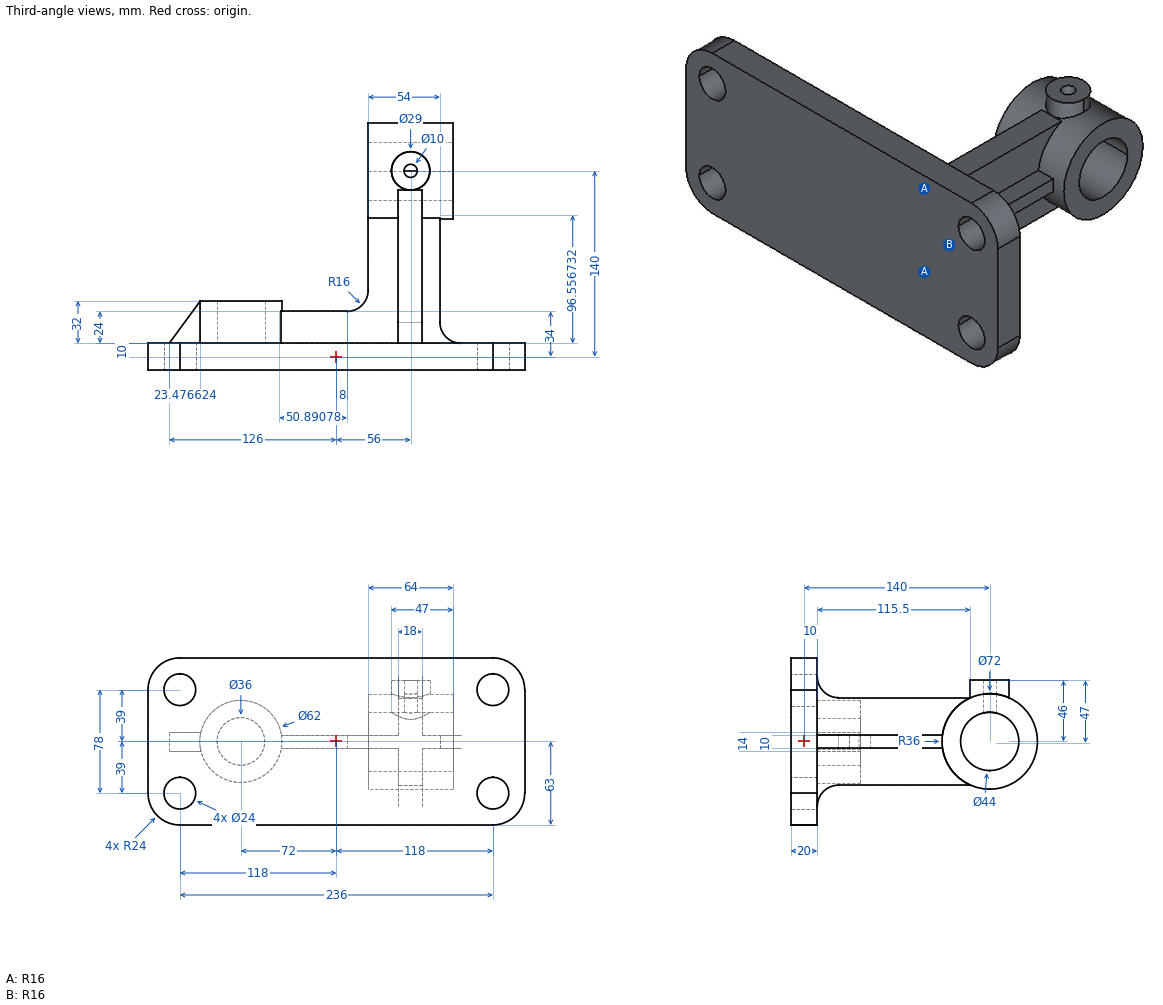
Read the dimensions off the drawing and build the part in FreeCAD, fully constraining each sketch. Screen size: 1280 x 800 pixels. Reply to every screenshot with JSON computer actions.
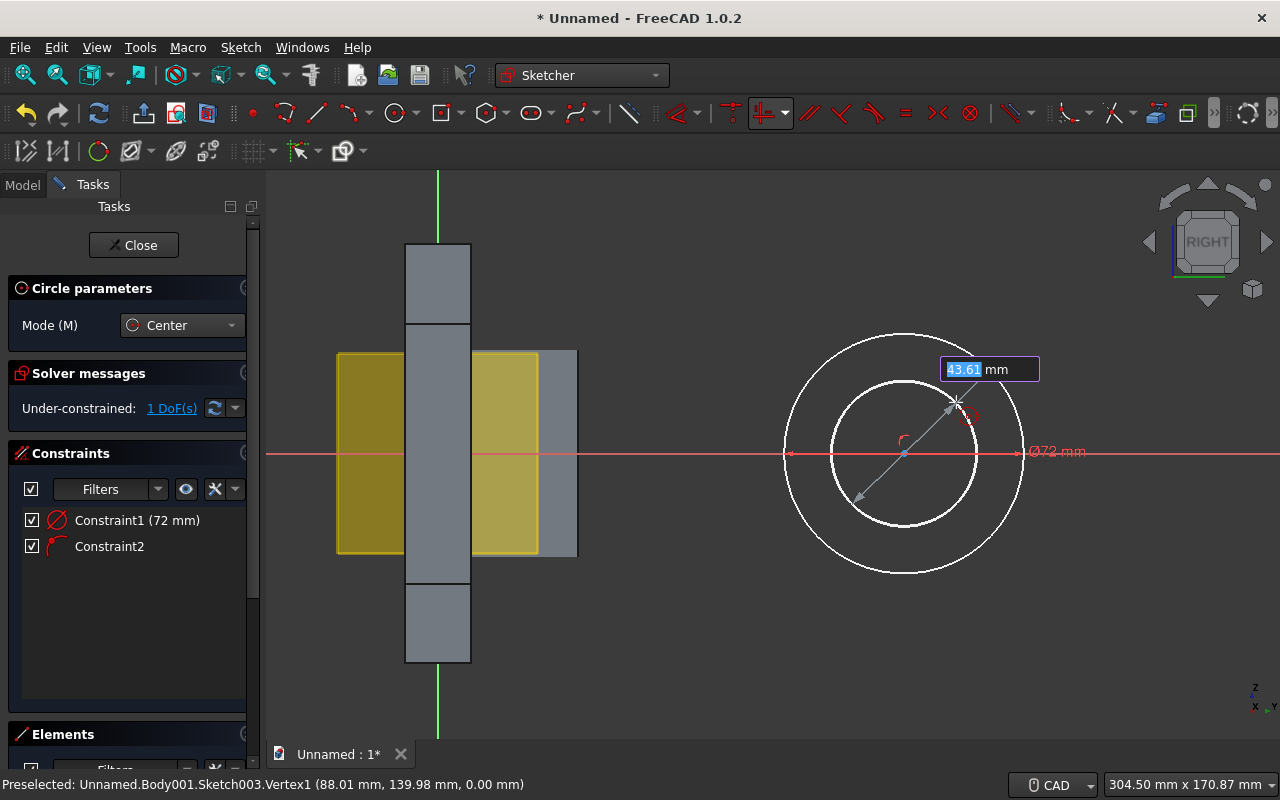
{"action": "type", "text": "44"}
{"action": "key", "text": "Return"}
{"action": "key", "text": "Escape"}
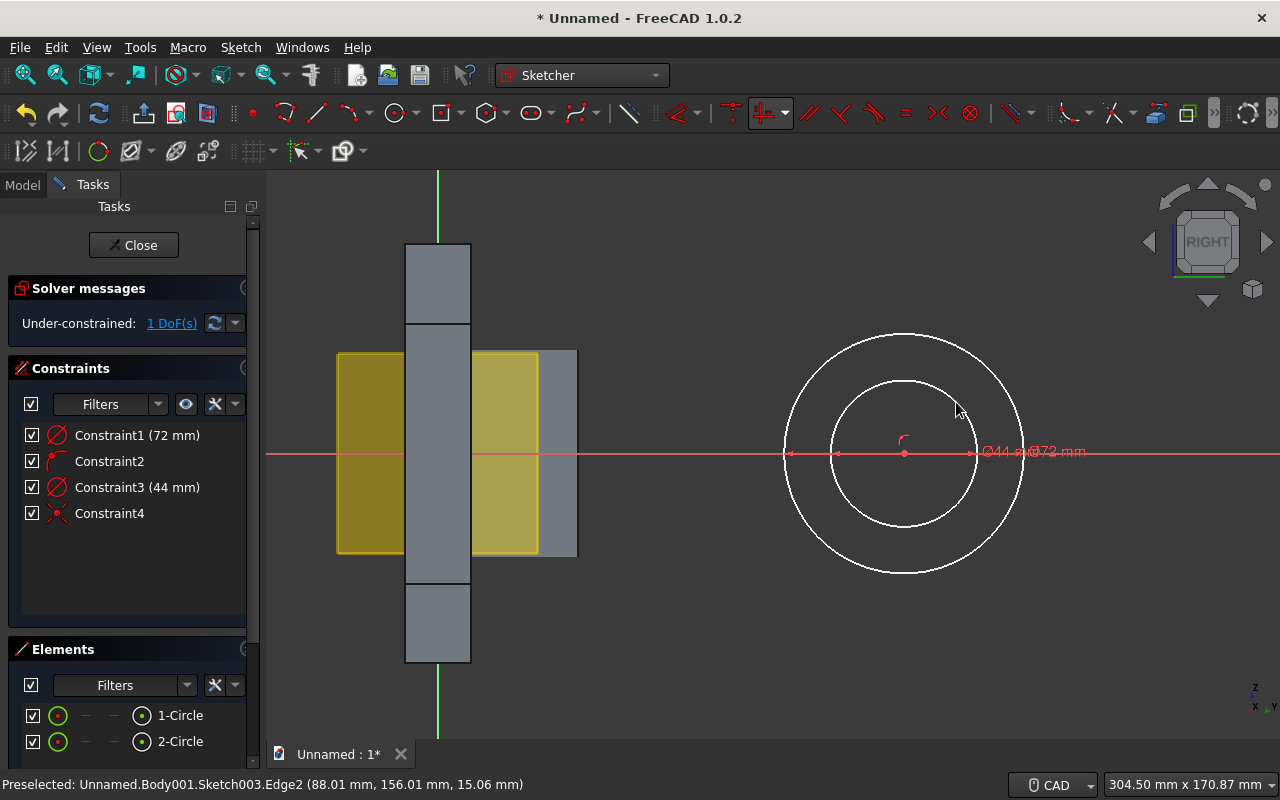
{"action": "left_click", "coordinate": [676, 114]}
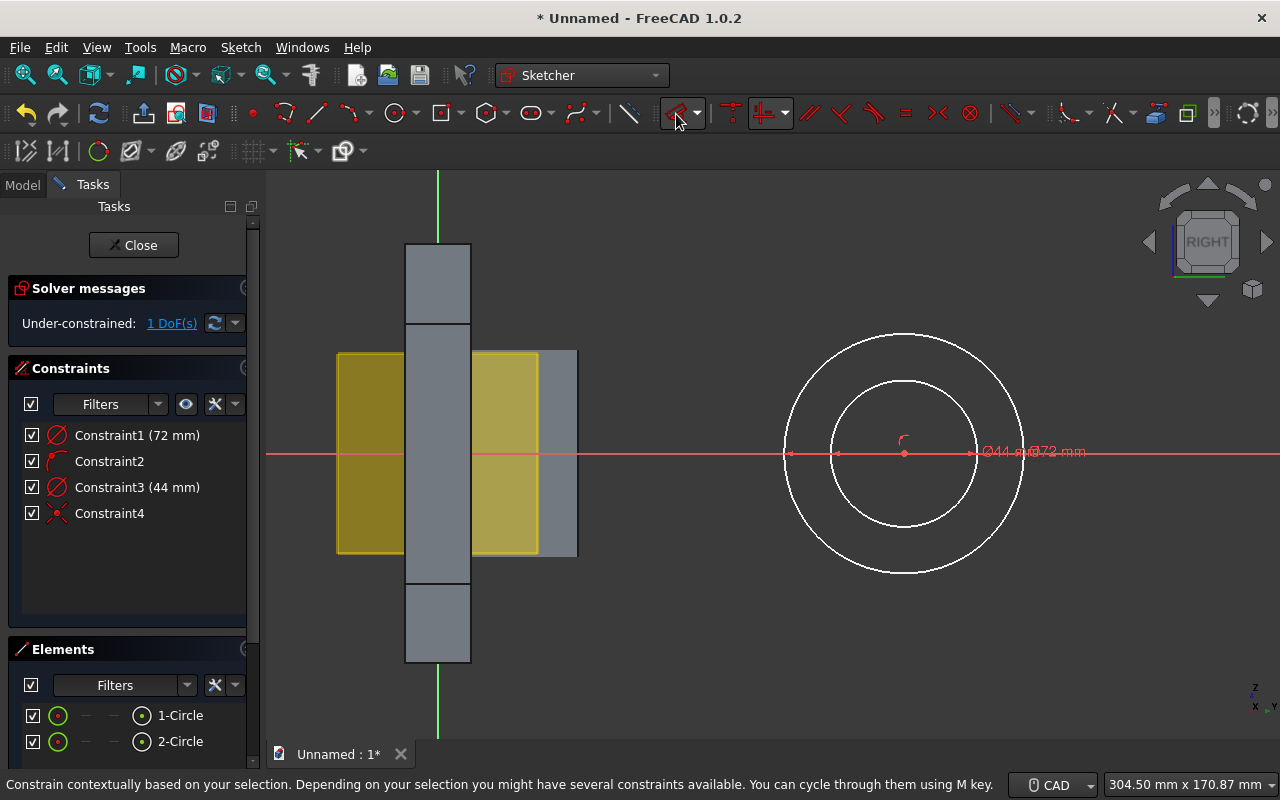
{"action": "left_click", "coordinate": [904, 454]}
{"action": "left_click", "coordinate": [671, 488]}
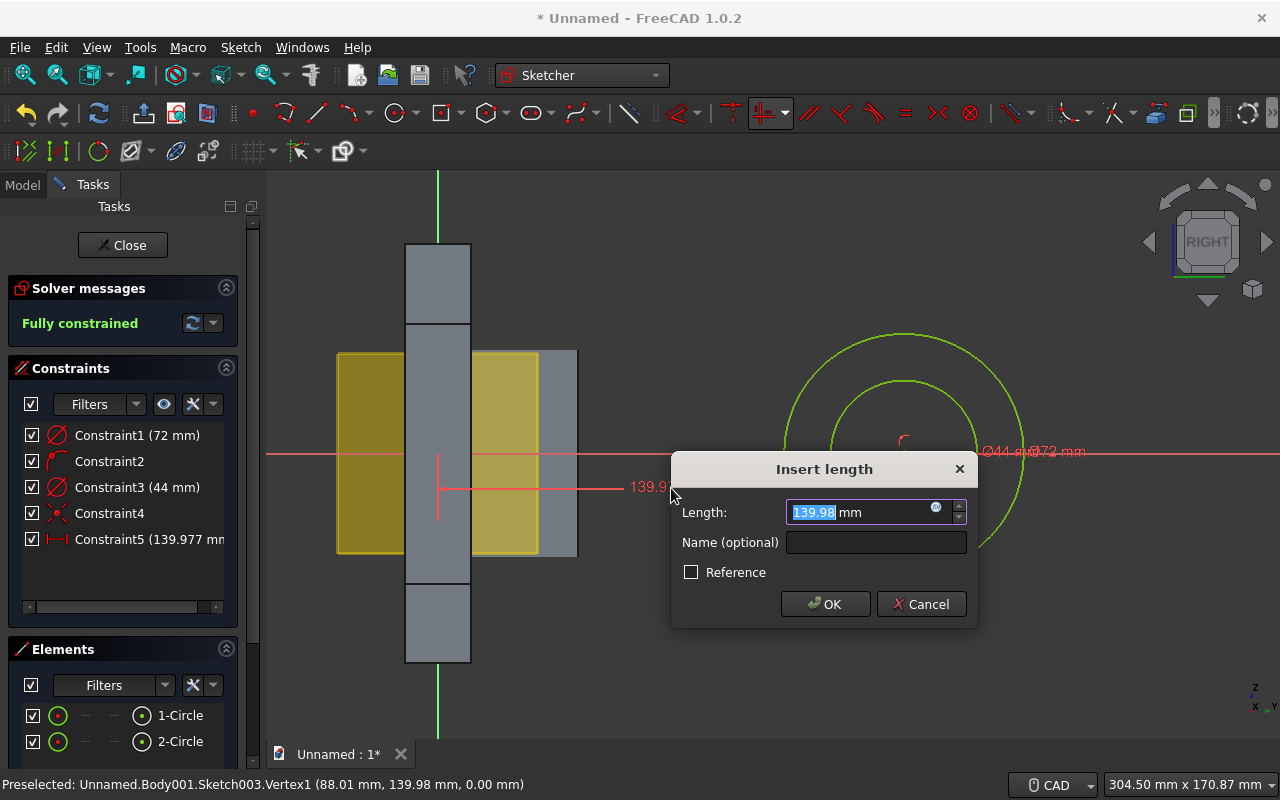
{"action": "type", "text": "140"}
{"action": "key", "text": "Return"}
{"action": "key", "text": "Escape"}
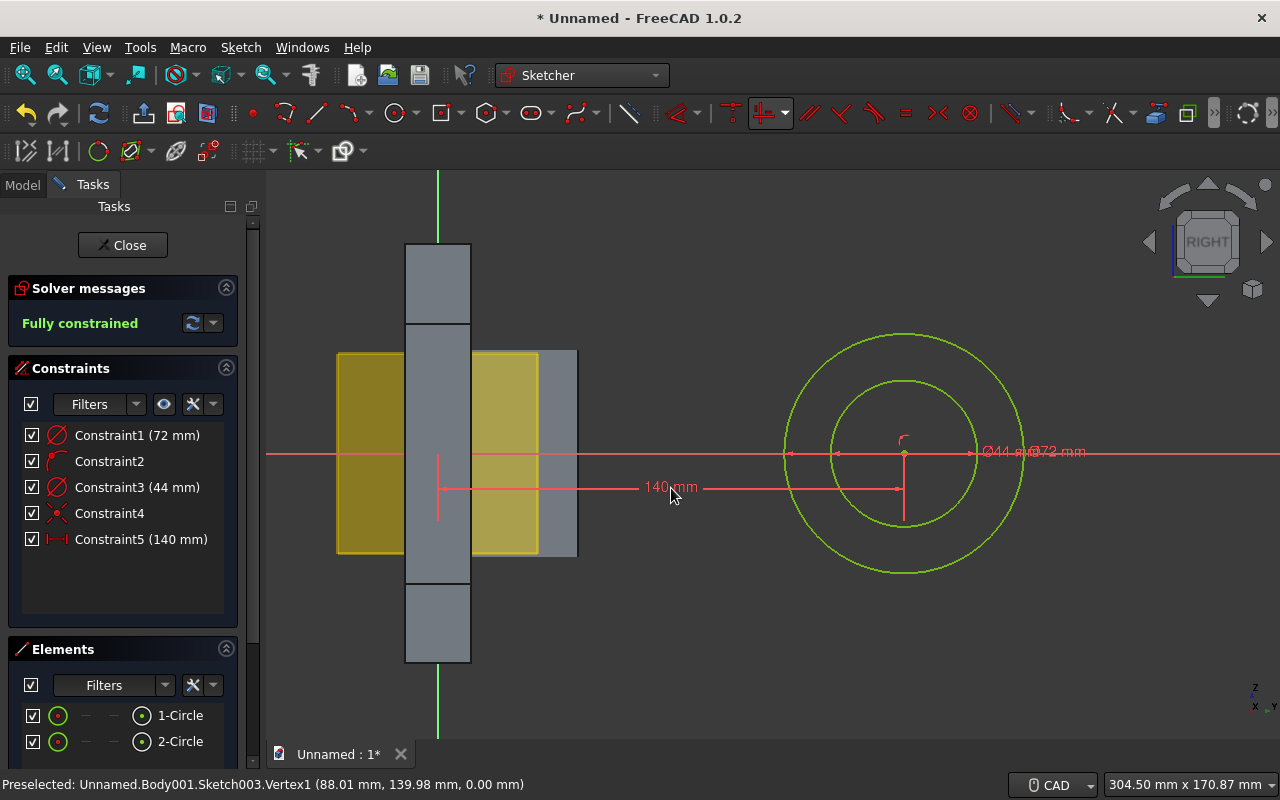
{"action": "left_click", "coordinate": [123, 245]}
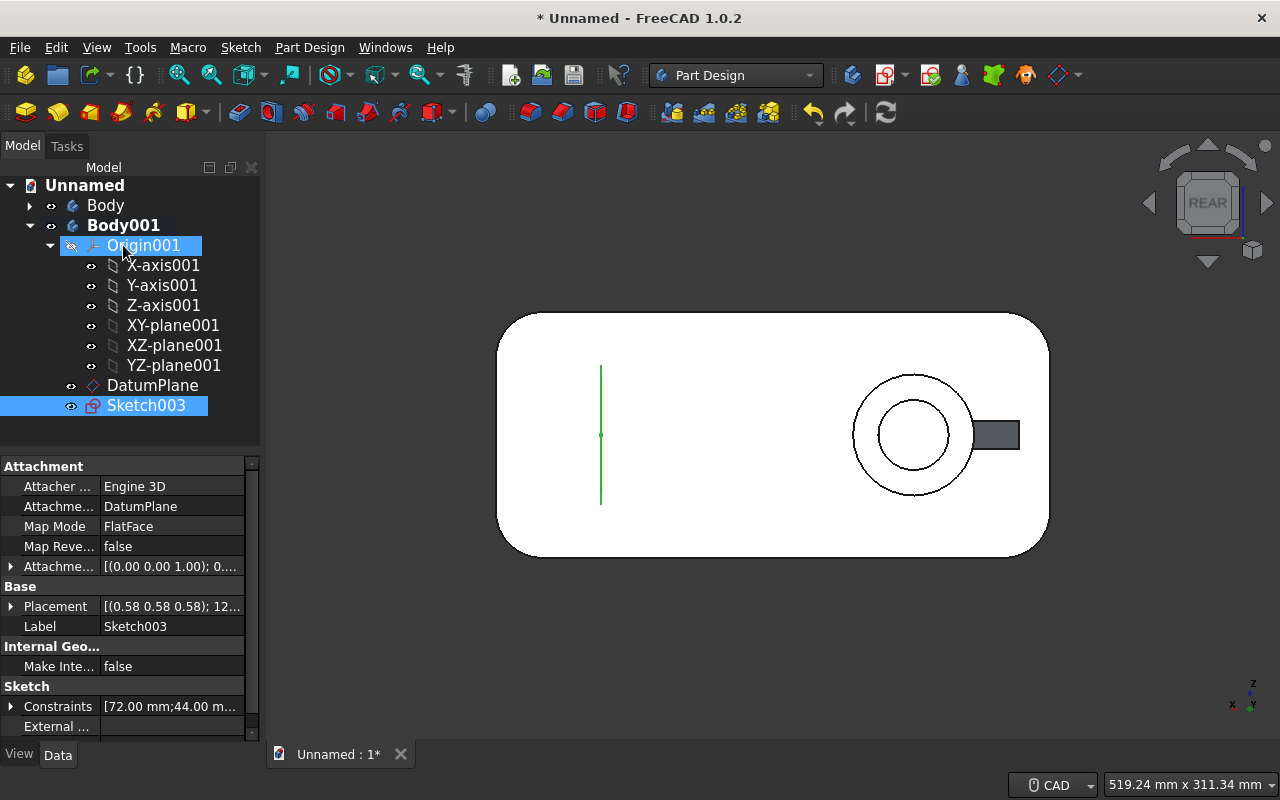
{"action": "left_click", "coordinate": [26, 112]}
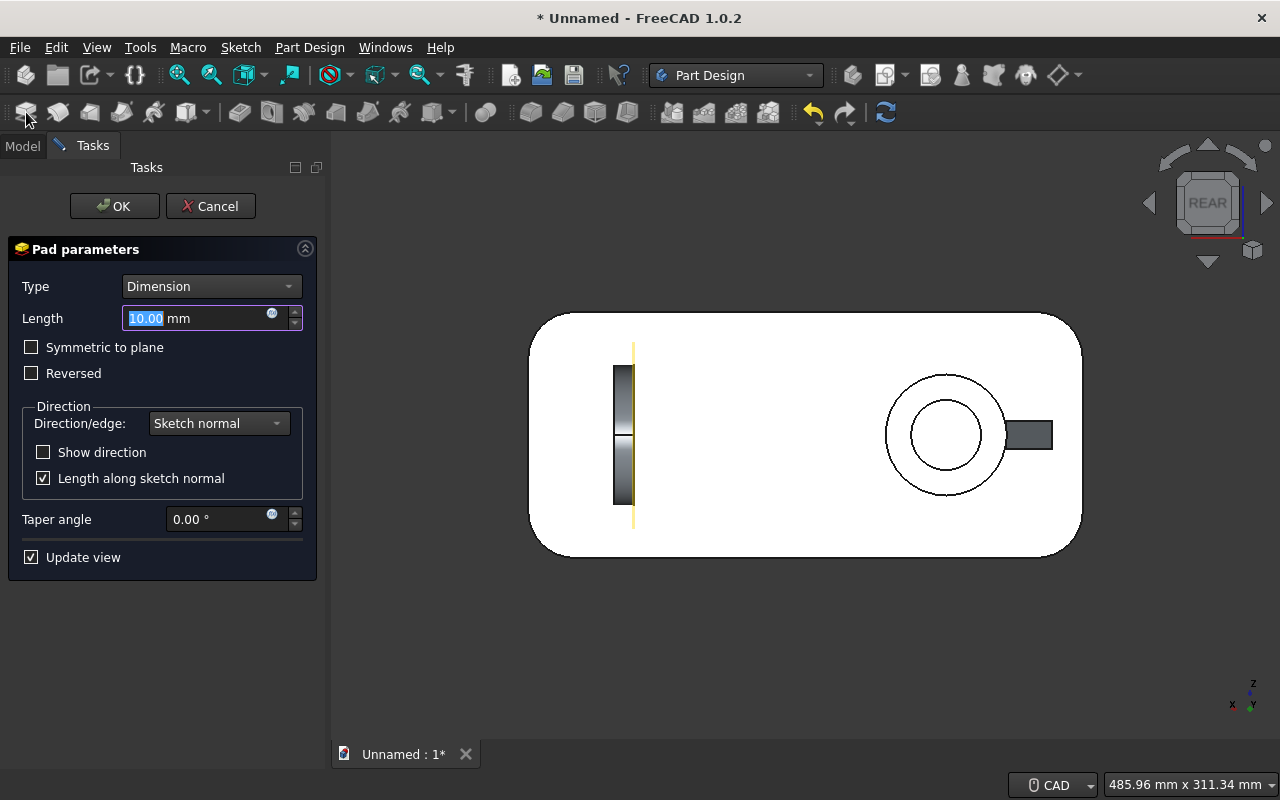
{"action": "type", "text": "64"}
{"action": "key", "text": "Tab"}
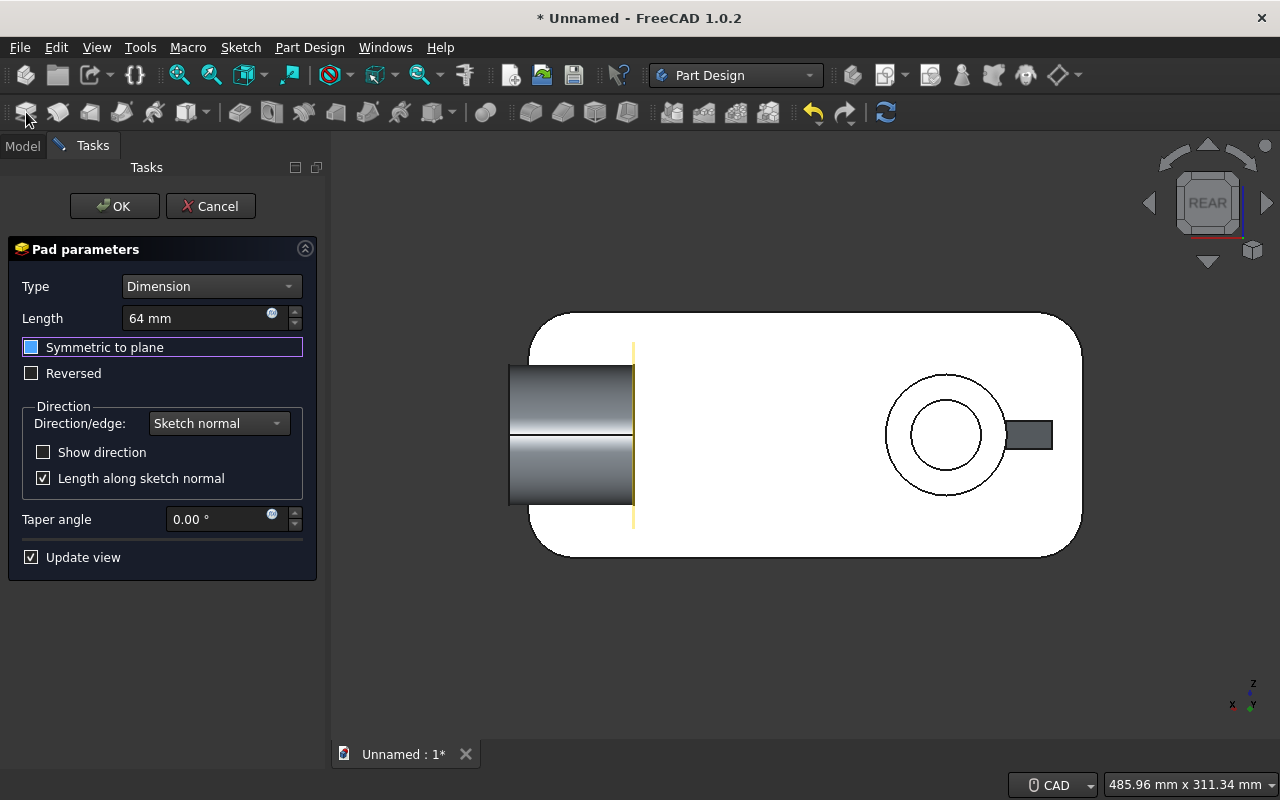
{"action": "left_click", "coordinate": [30, 373]}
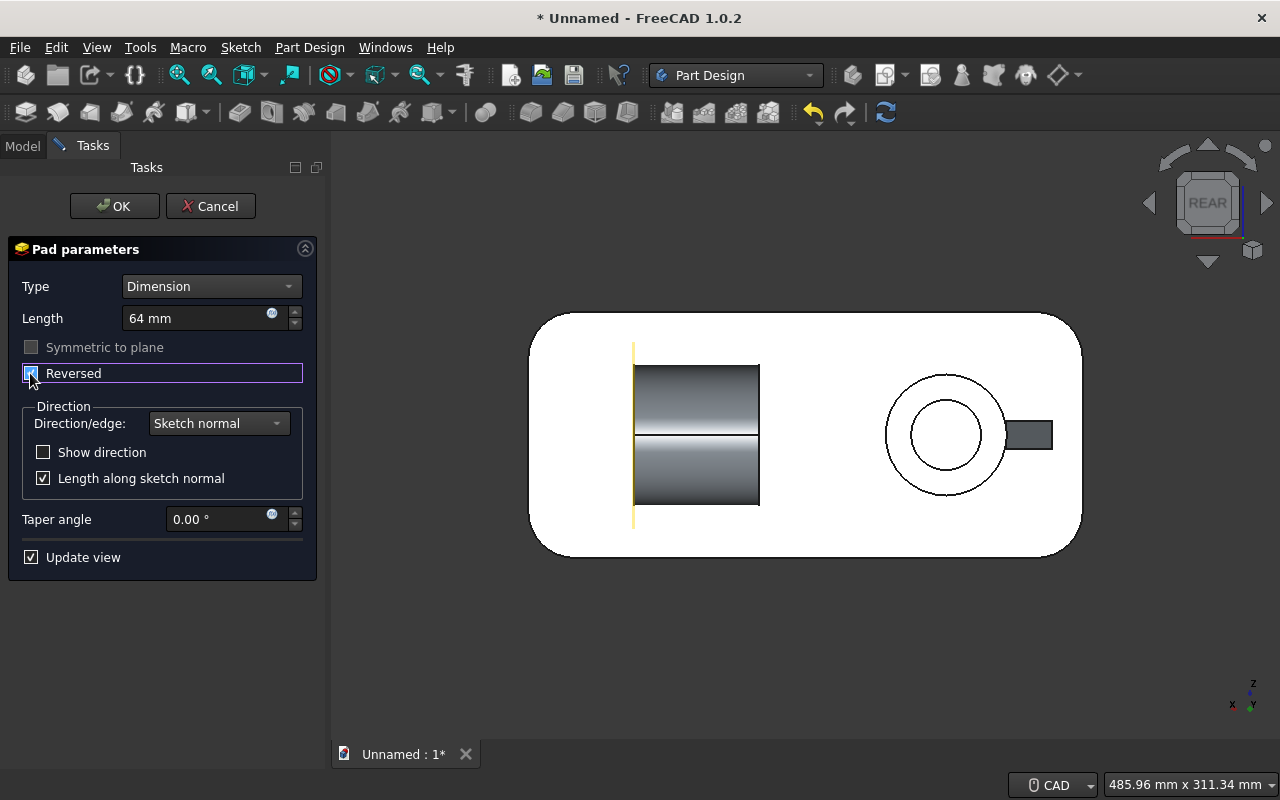
{"action": "left_click", "coordinate": [115, 206]}